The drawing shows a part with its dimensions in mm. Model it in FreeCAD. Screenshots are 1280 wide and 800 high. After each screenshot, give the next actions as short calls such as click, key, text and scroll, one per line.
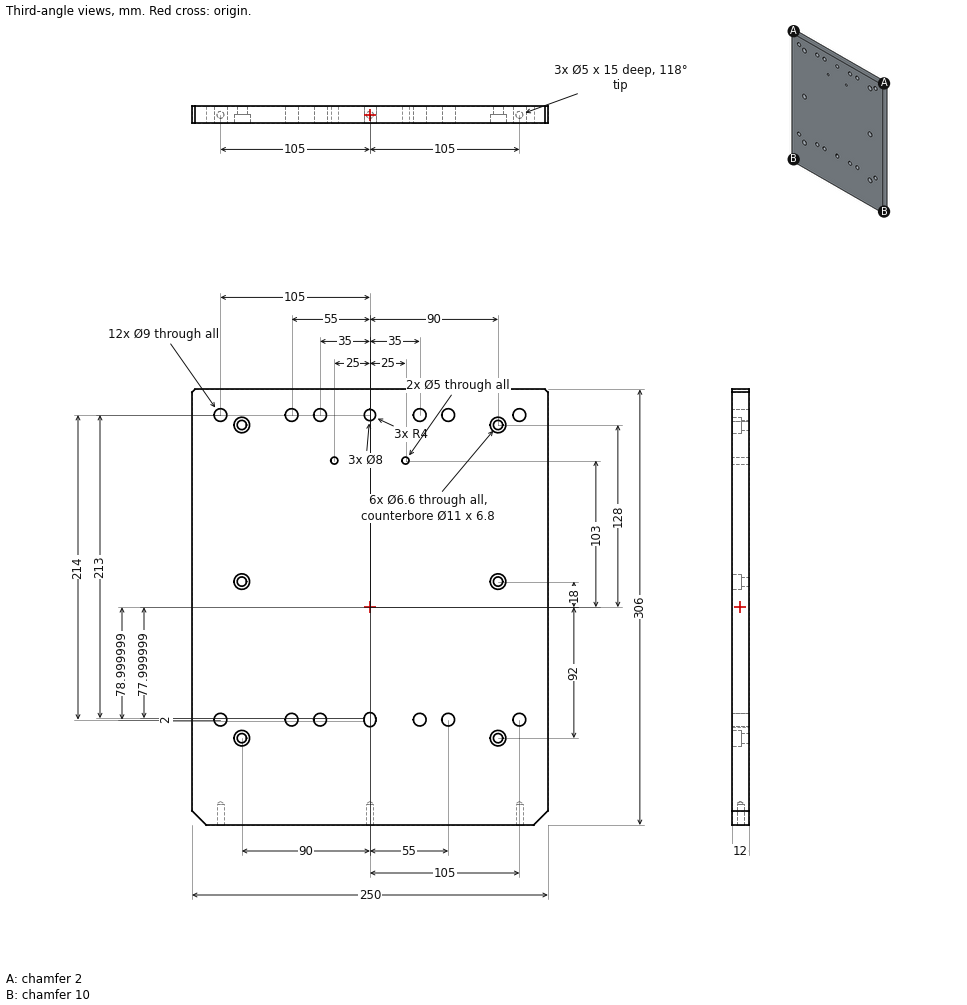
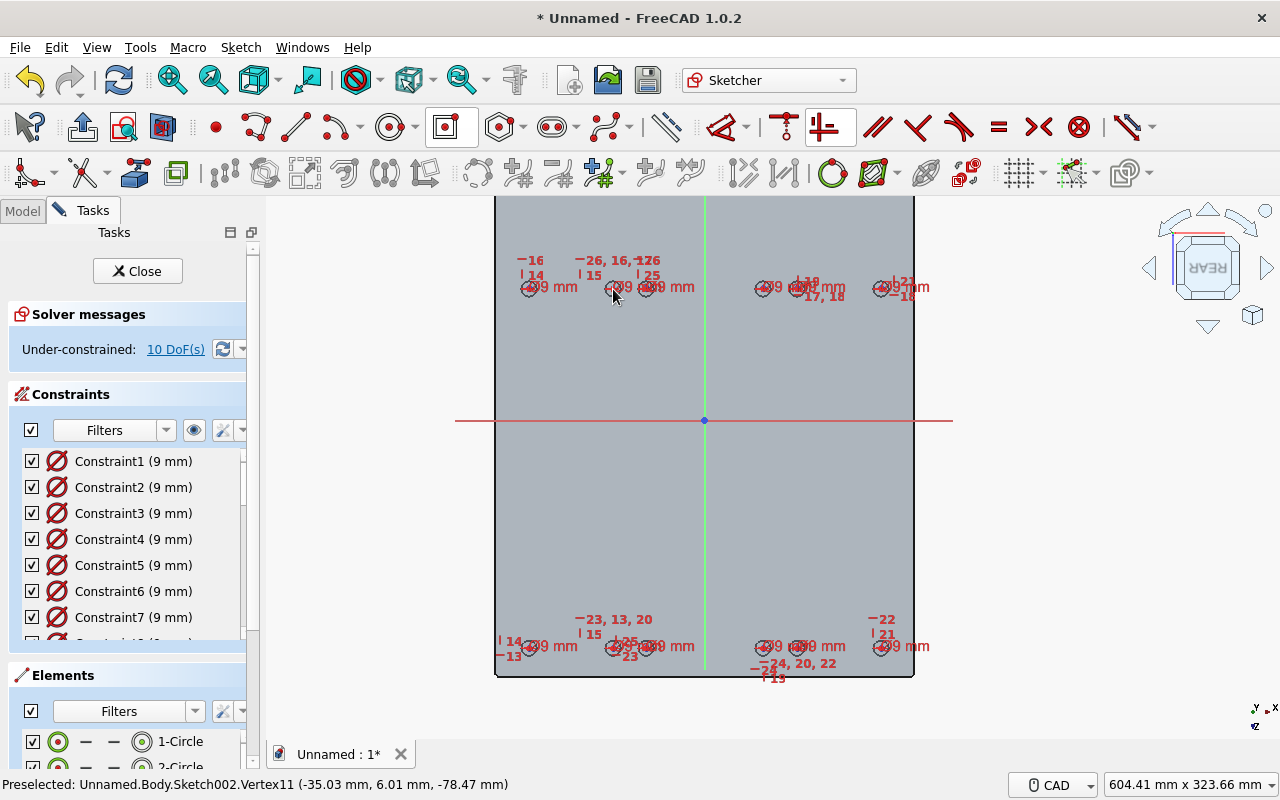
click(763, 648)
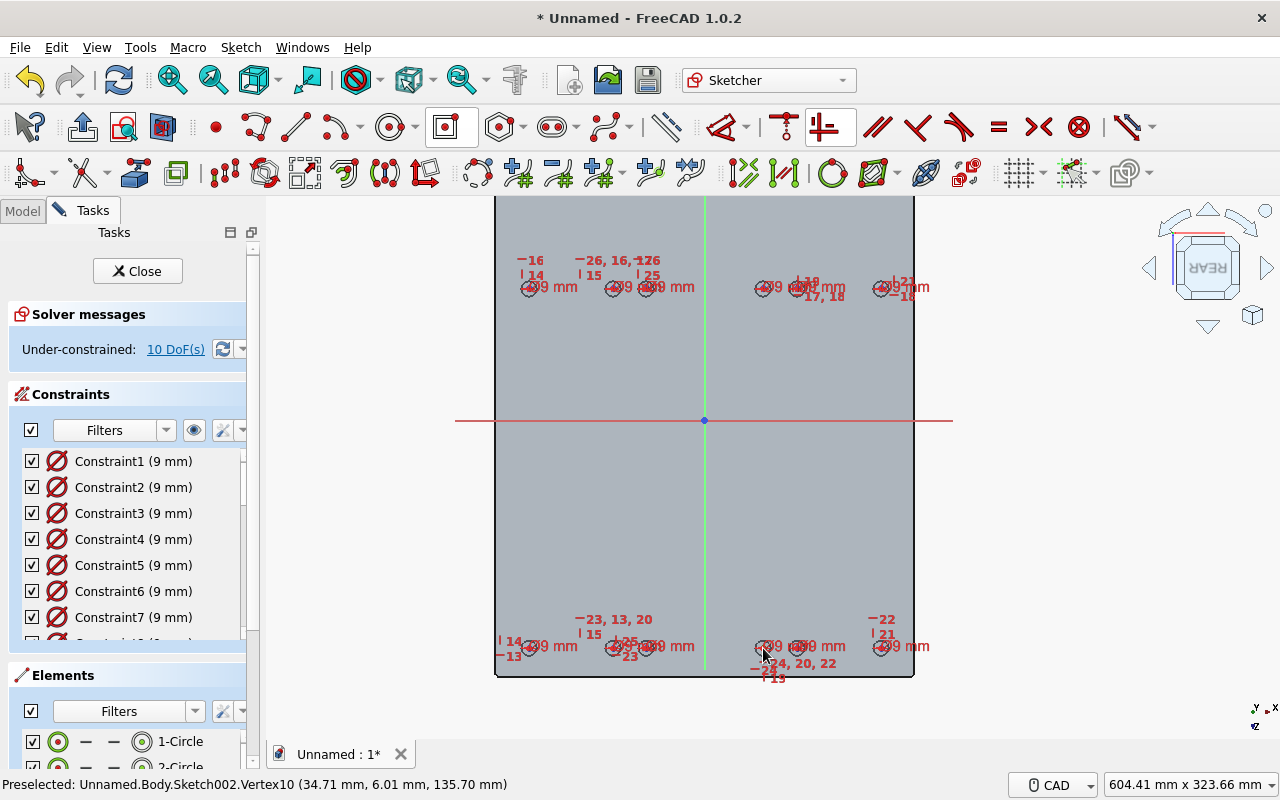
click(763, 289)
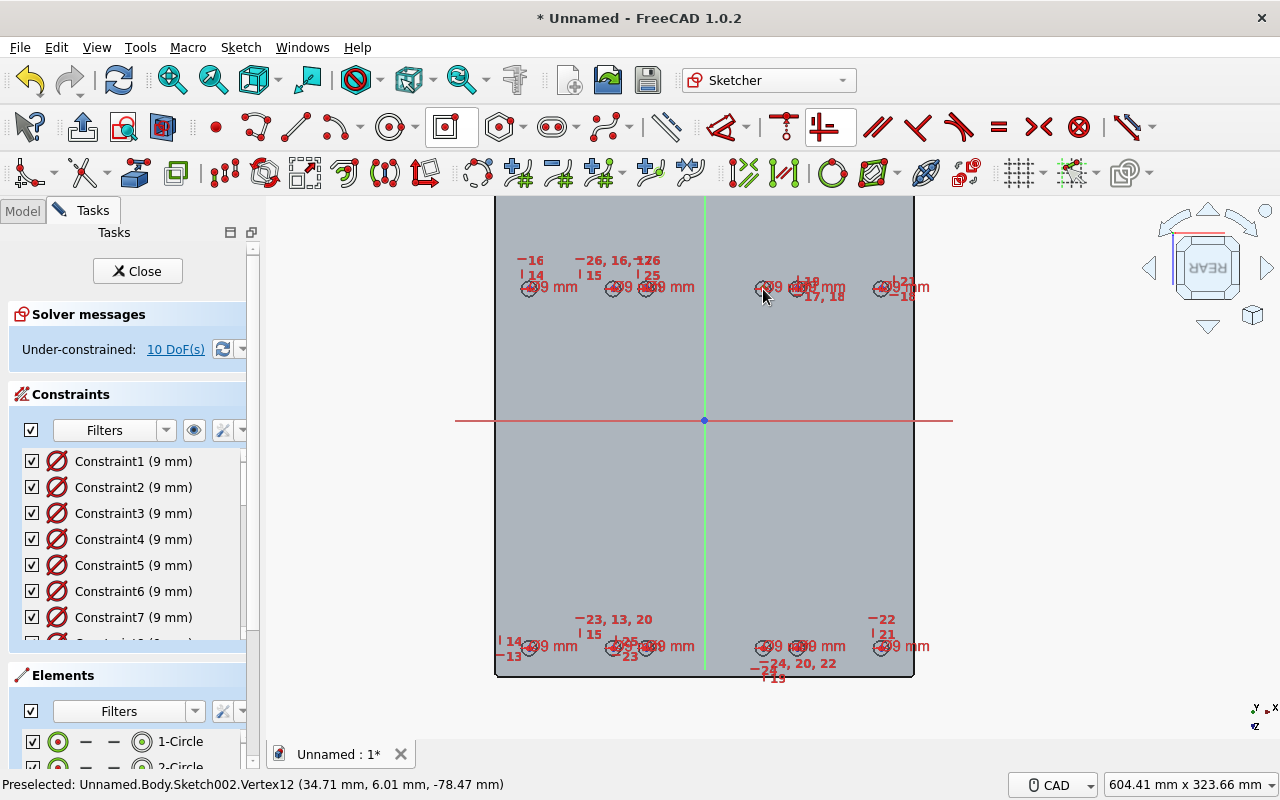
click(850, 128)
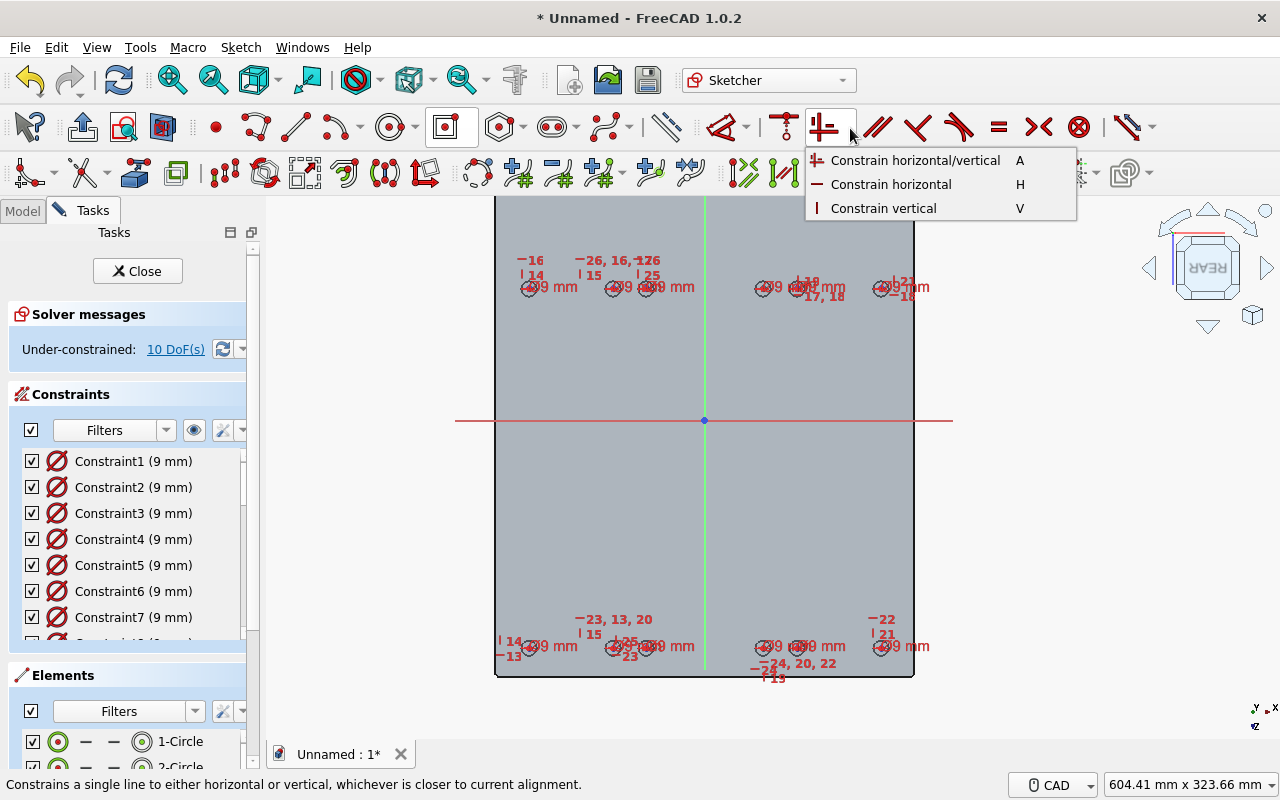
click(941, 208)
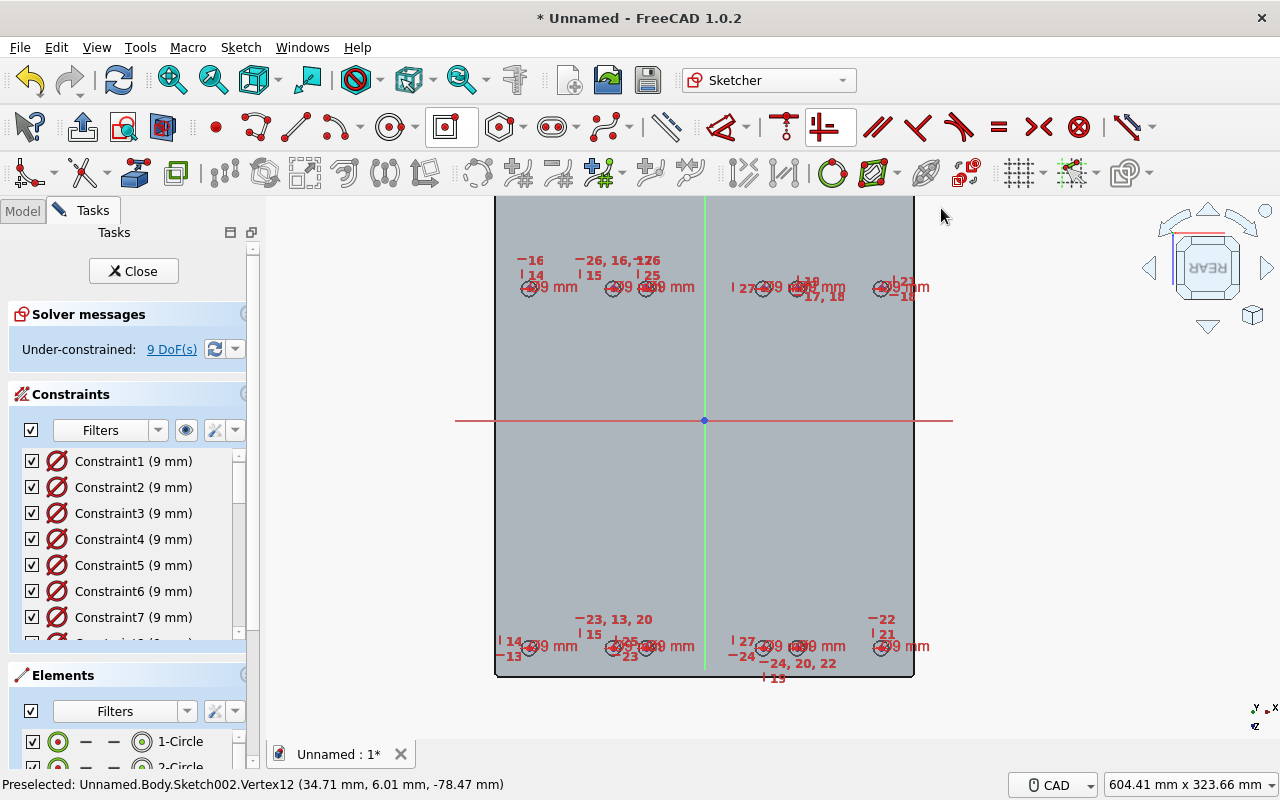
click(797, 289)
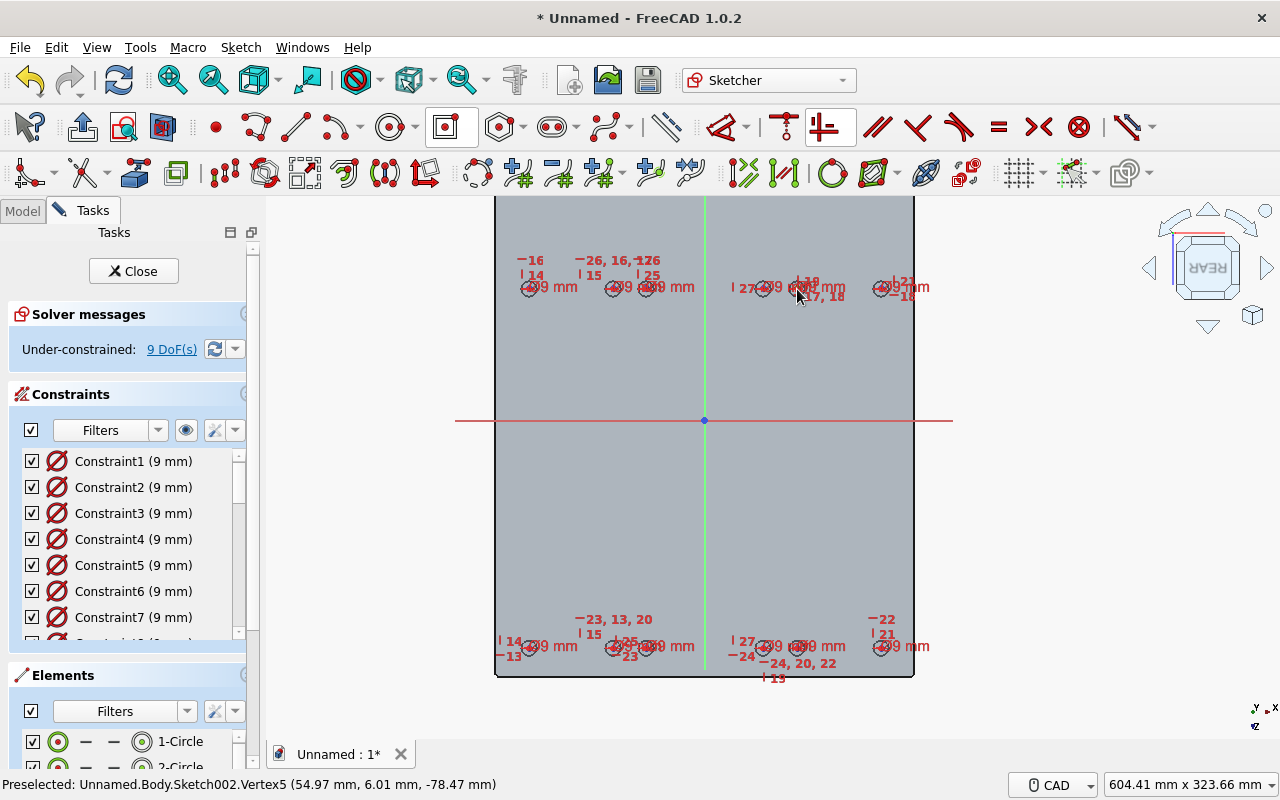
click(763, 289)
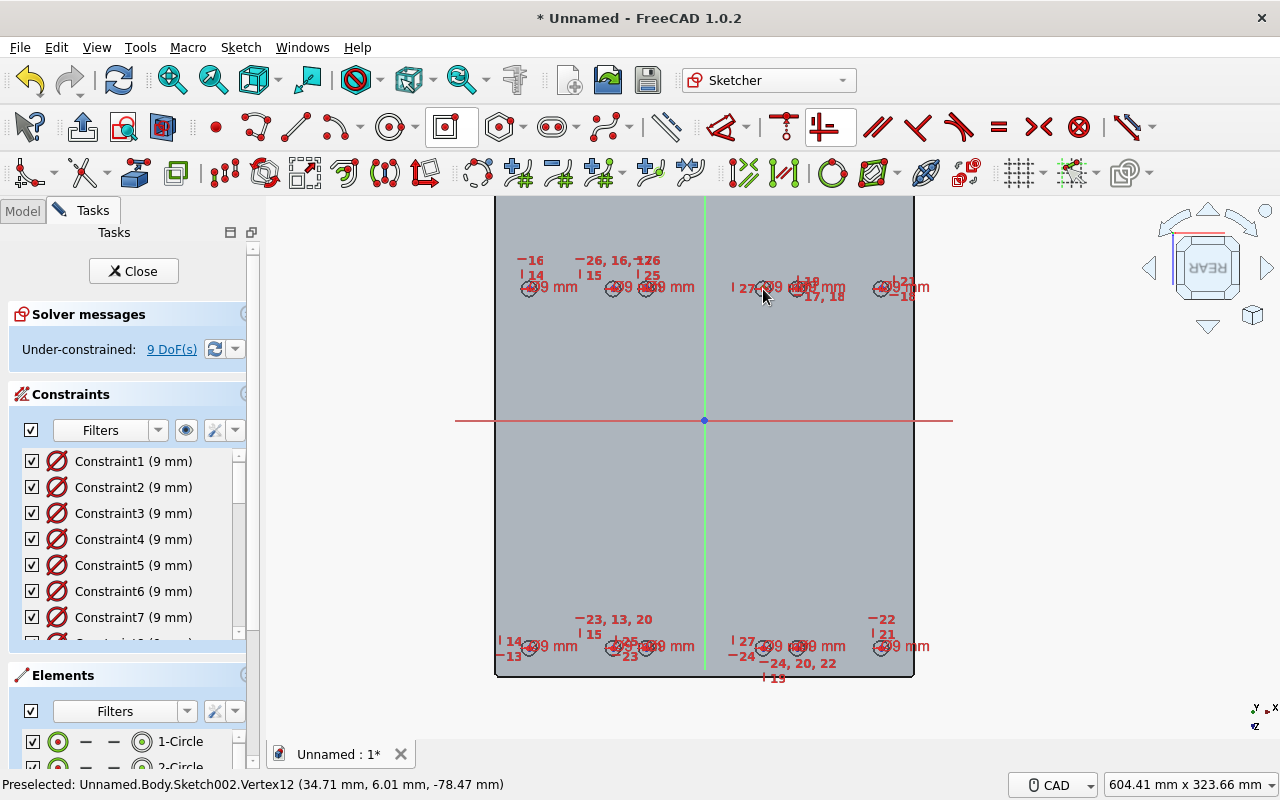
key(h)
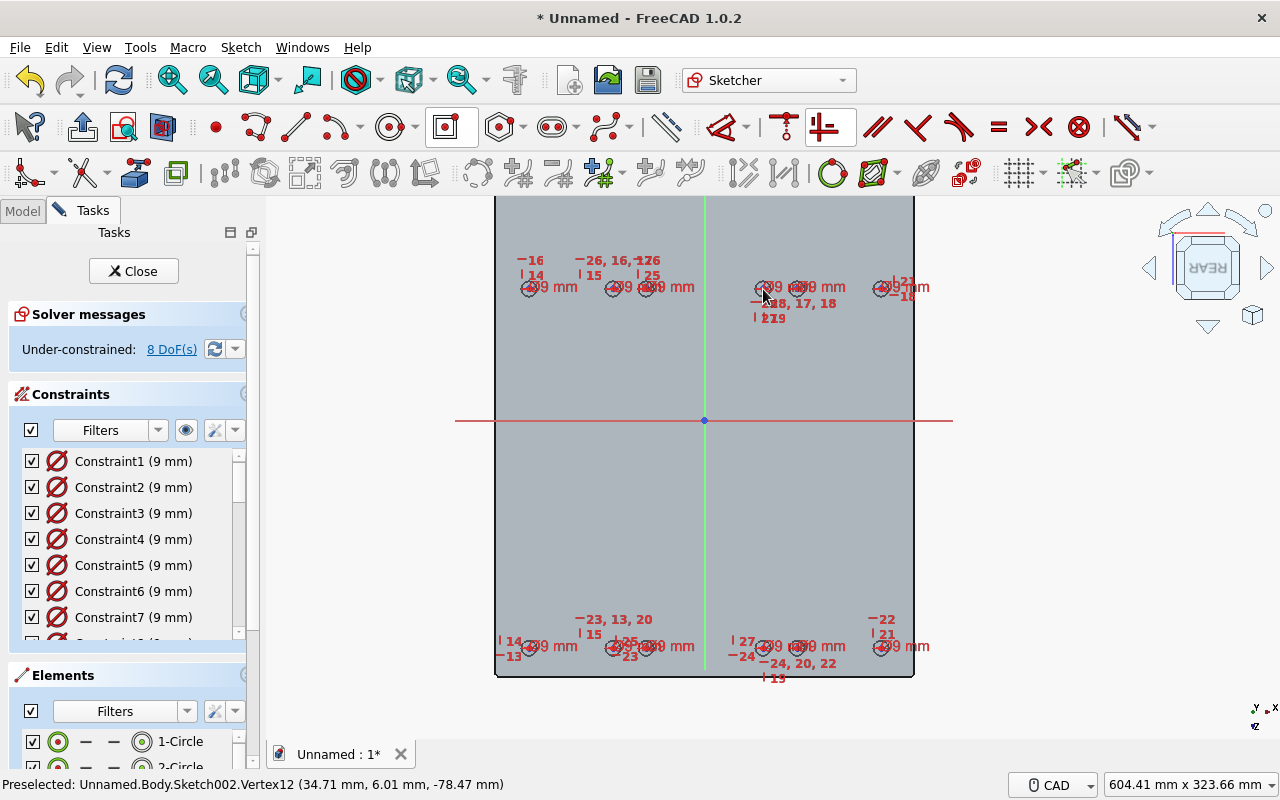
click(722, 128)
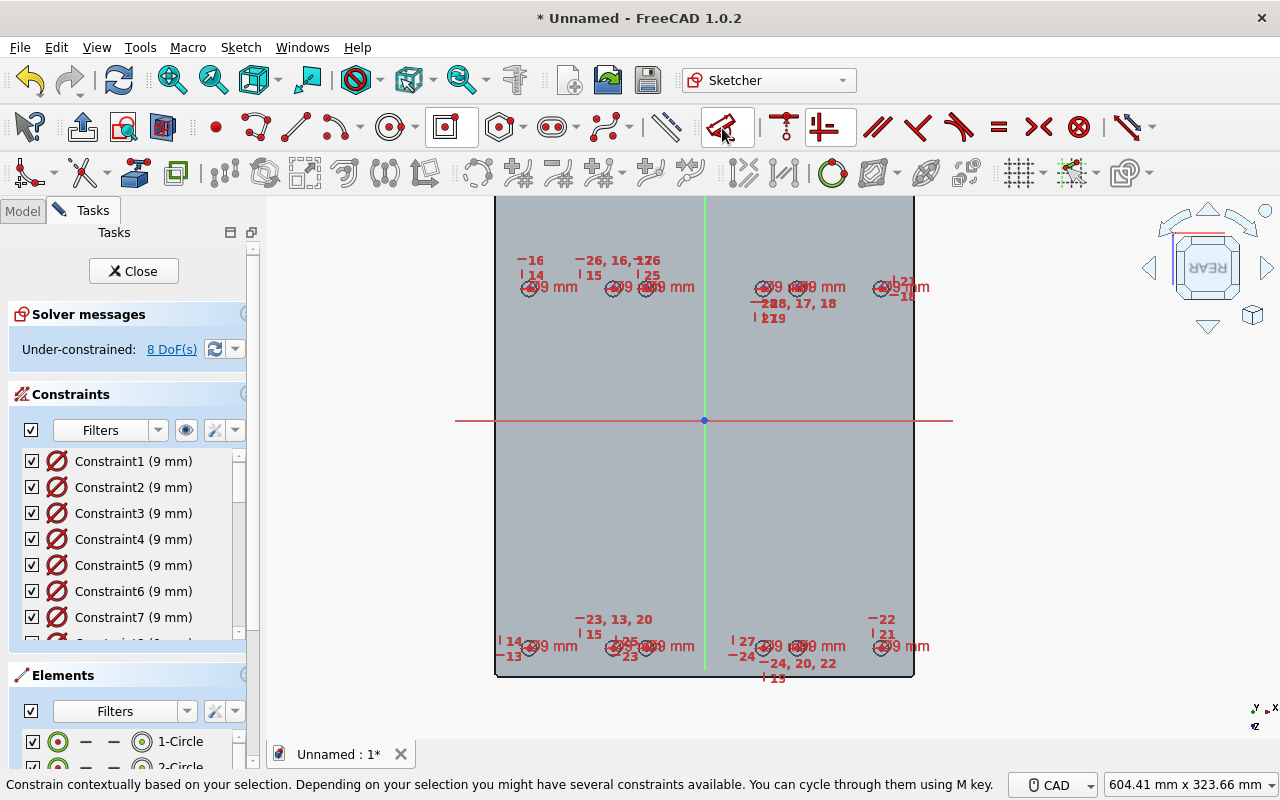
click(613, 648)
click(659, 682)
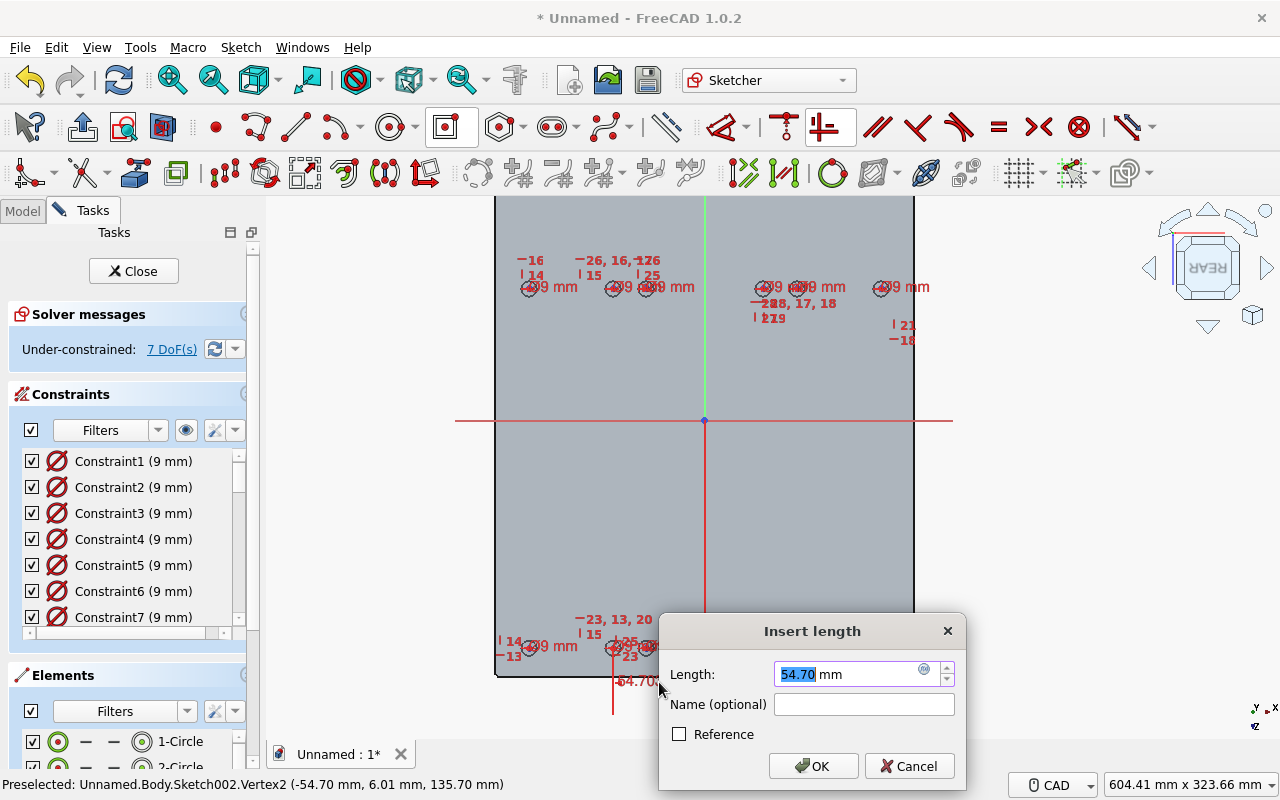
text(55)
key(Return)